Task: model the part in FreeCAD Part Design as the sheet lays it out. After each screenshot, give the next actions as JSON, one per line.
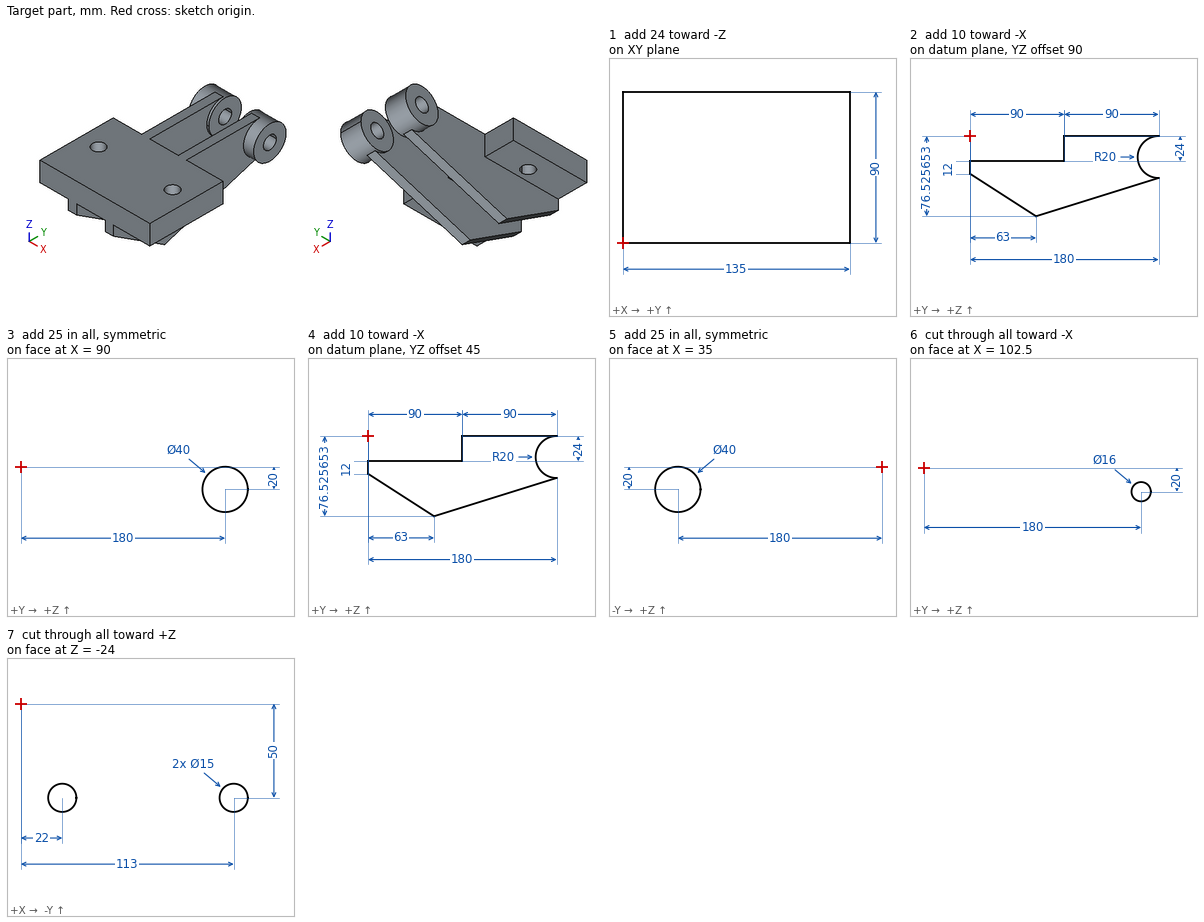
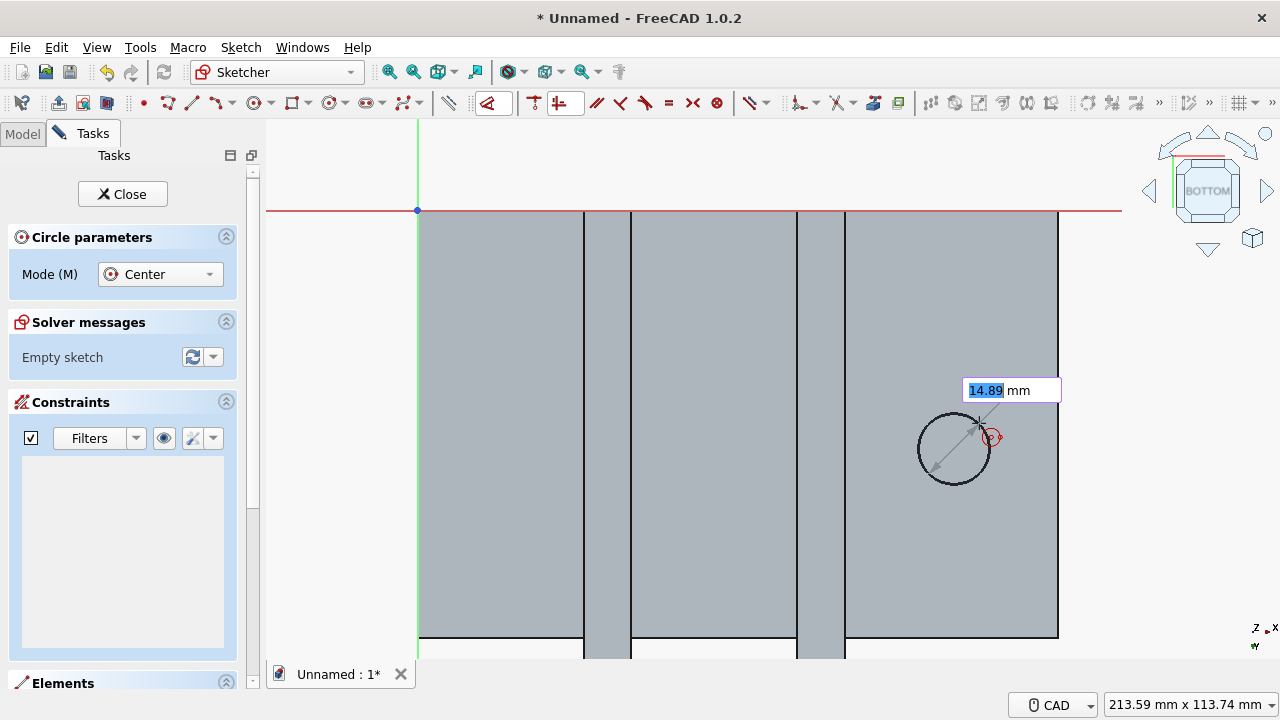
{"action": "type", "text": "15"}
{"action": "key", "text": "Return"}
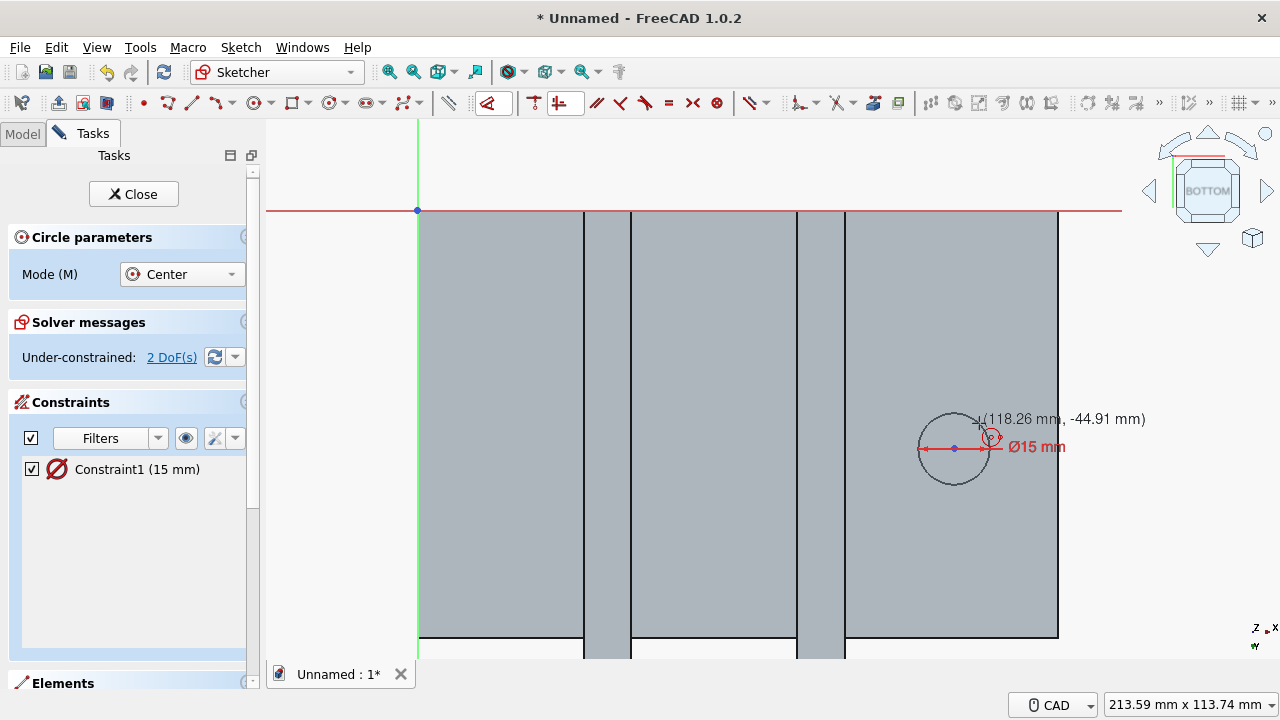
{"action": "left_click", "coordinate": [522, 448]}
{"action": "mouse_move", "coordinate": [547, 423]}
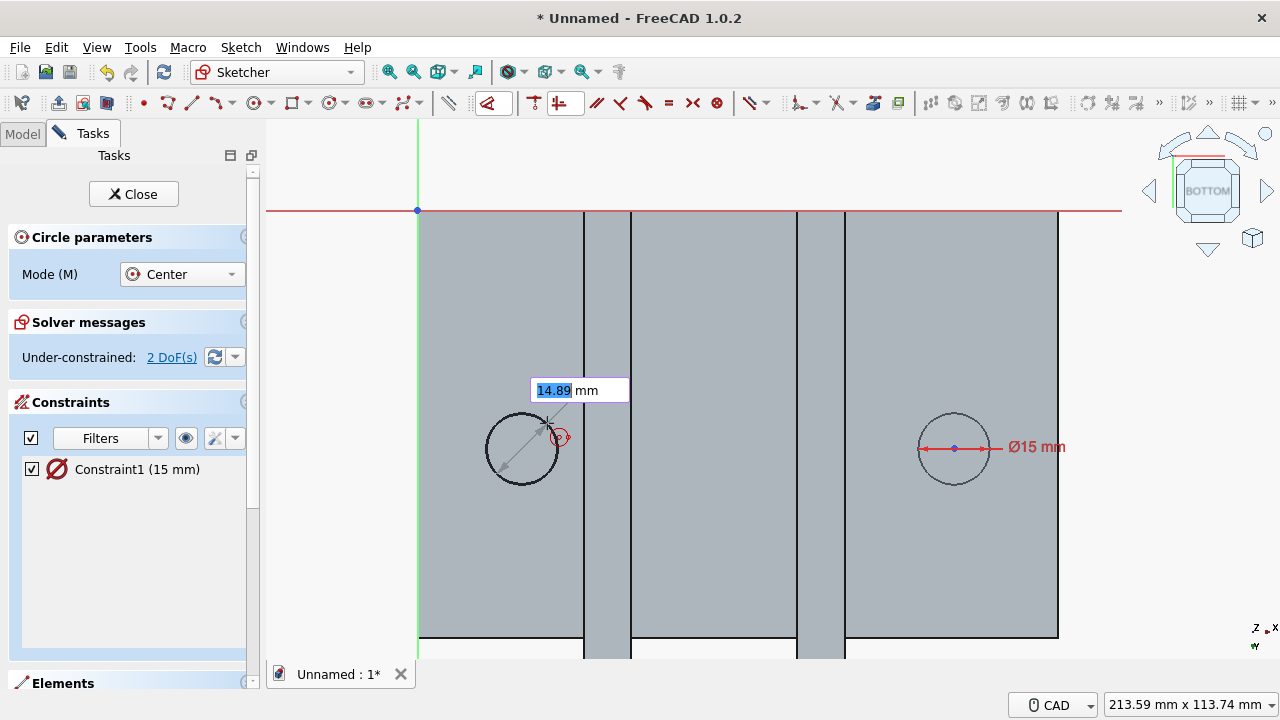
{"action": "type", "text": "15"}
{"action": "key", "text": "Return"}
{"action": "key", "text": "Escape"}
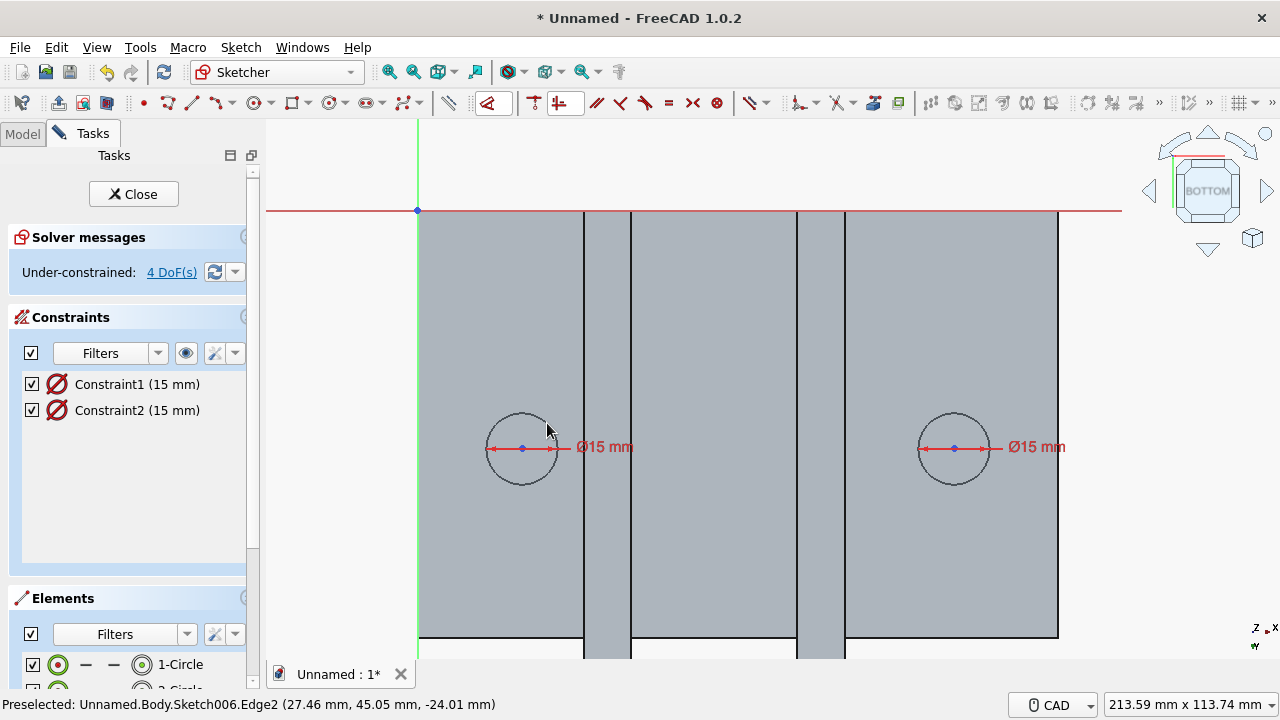
{"action": "left_click", "coordinate": [954, 449]}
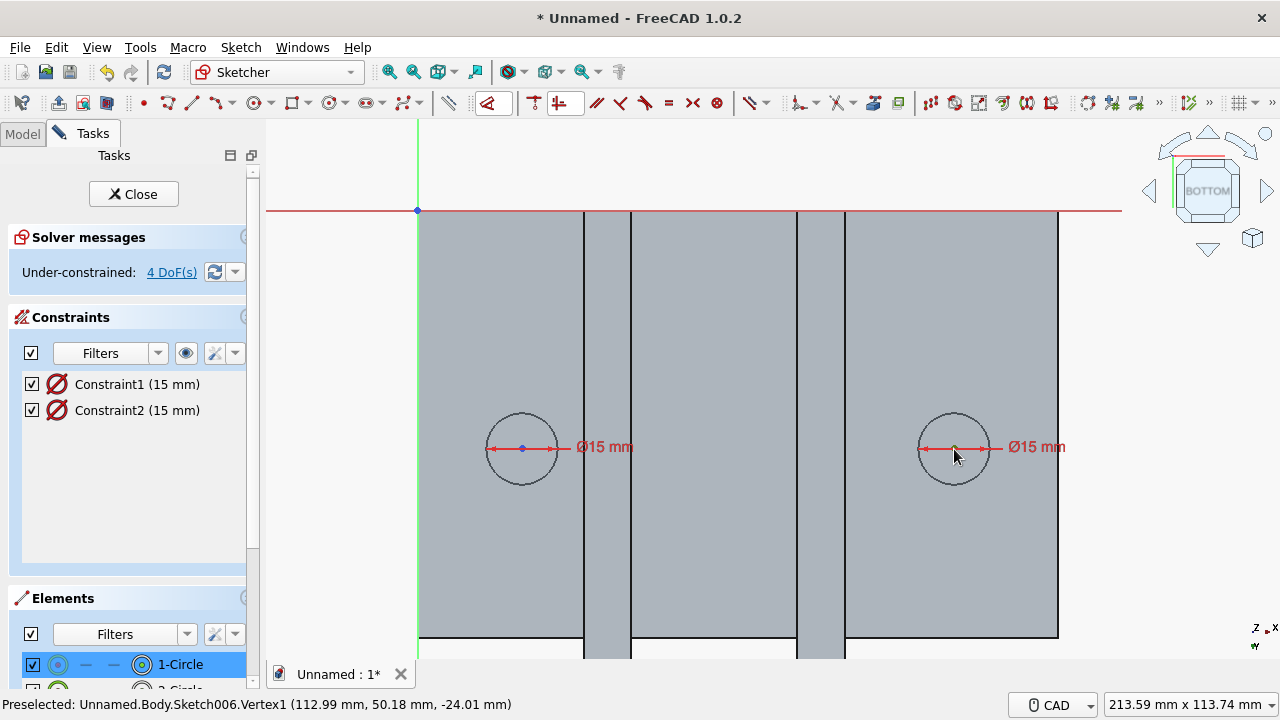
{"action": "left_click", "coordinate": [522, 449]}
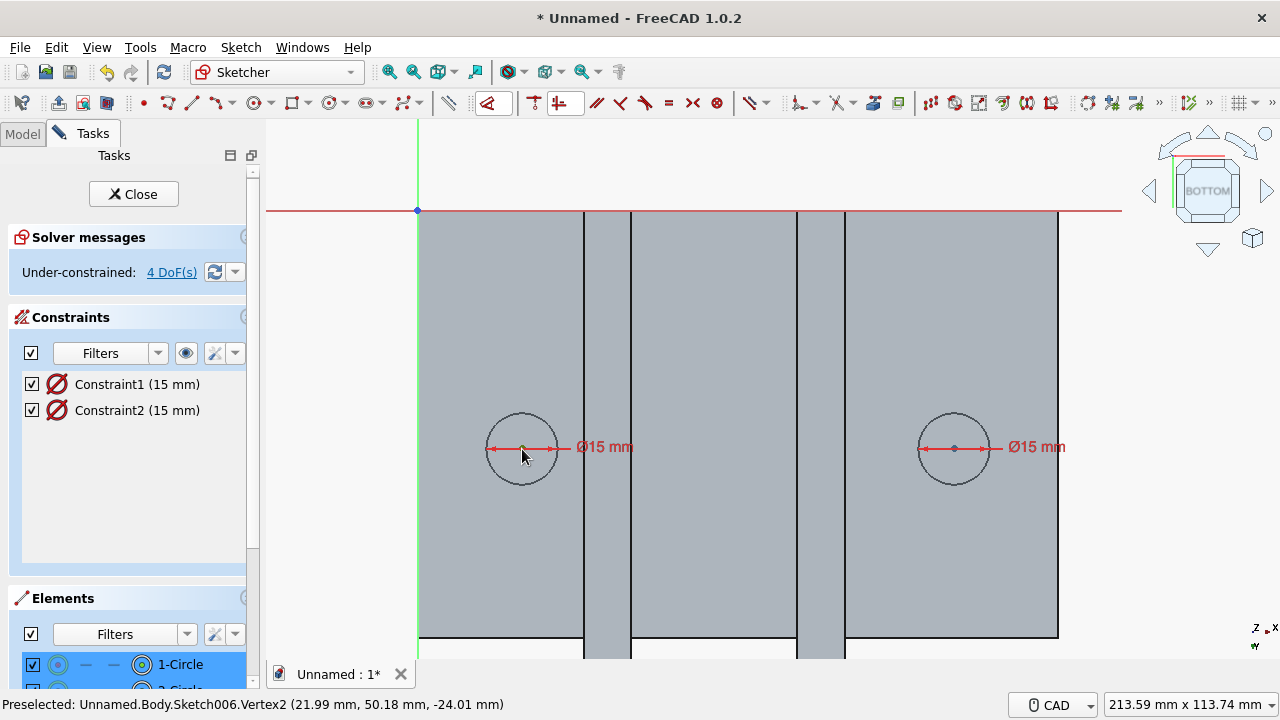
{"action": "left_click", "coordinate": [578, 104]}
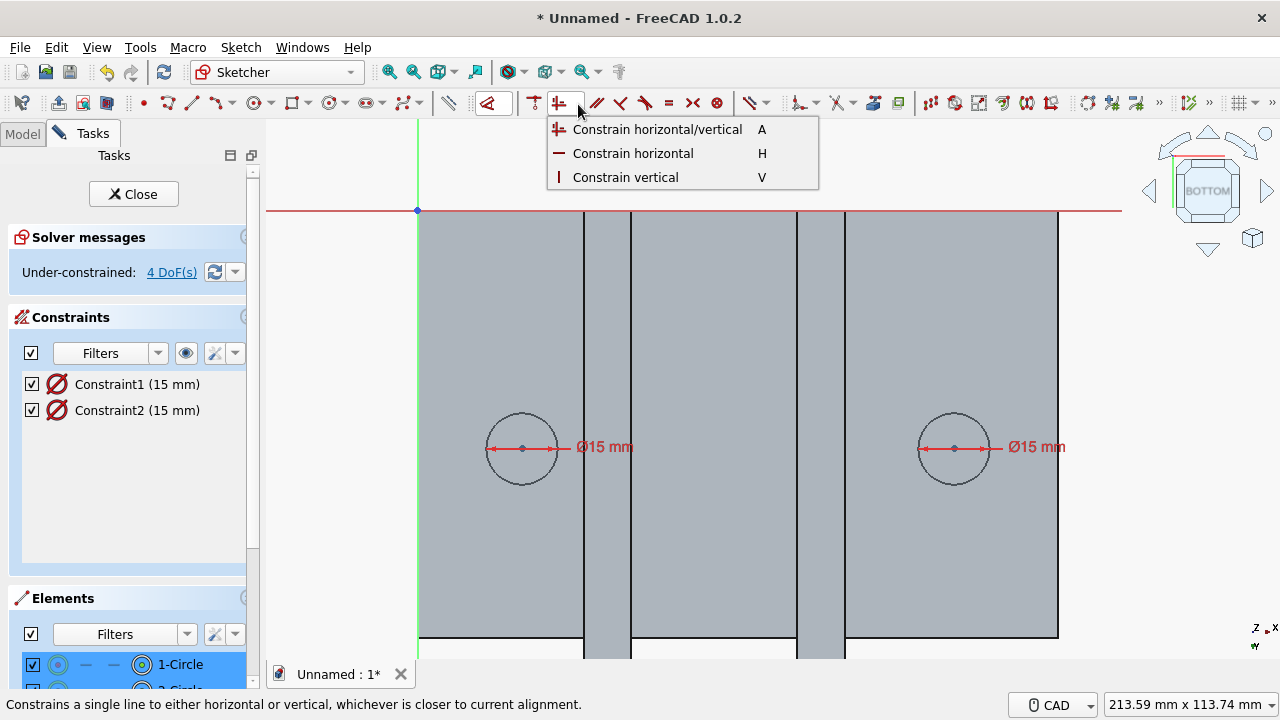
{"action": "left_click", "coordinate": [683, 153]}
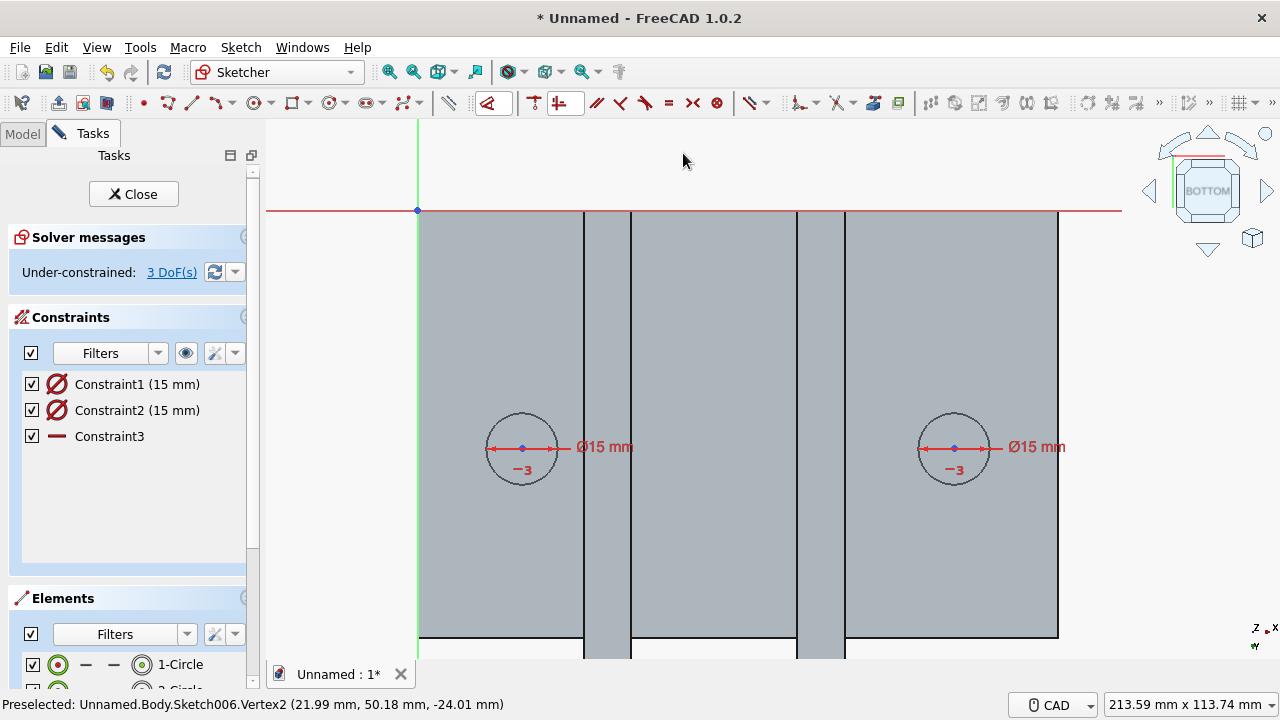
{"action": "left_click", "coordinate": [954, 449]}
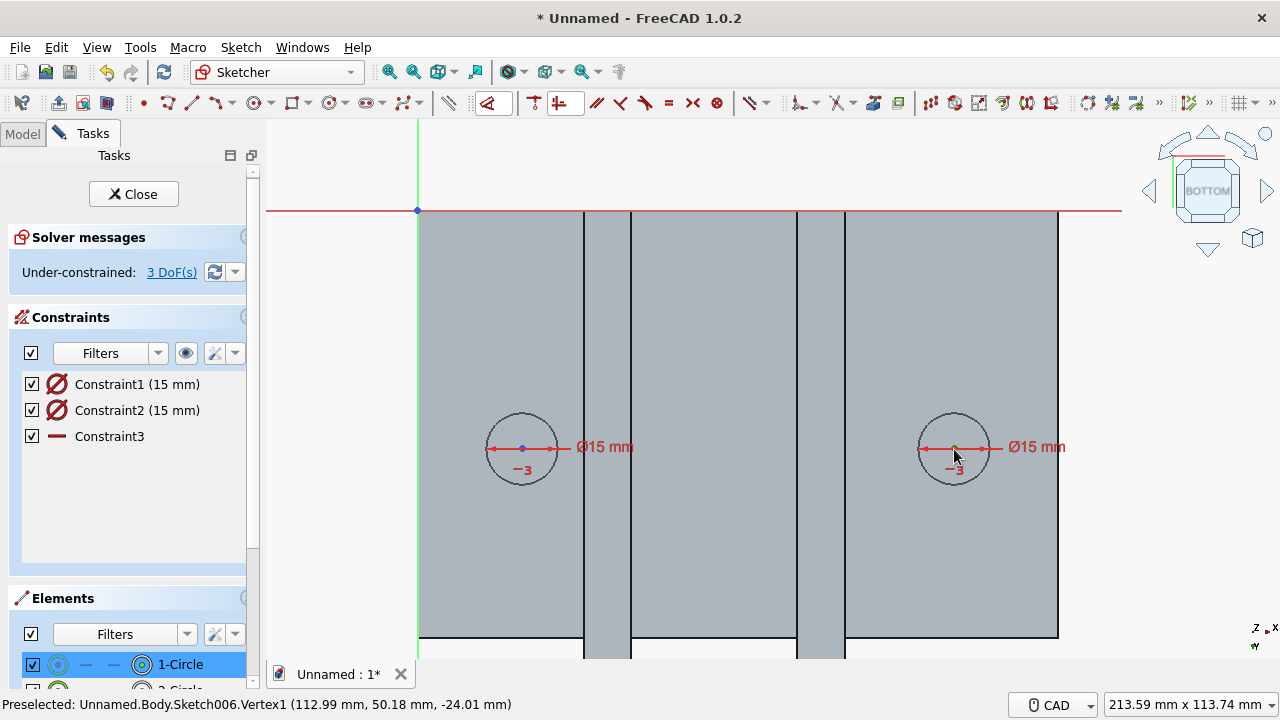
{"action": "key", "text": "i"}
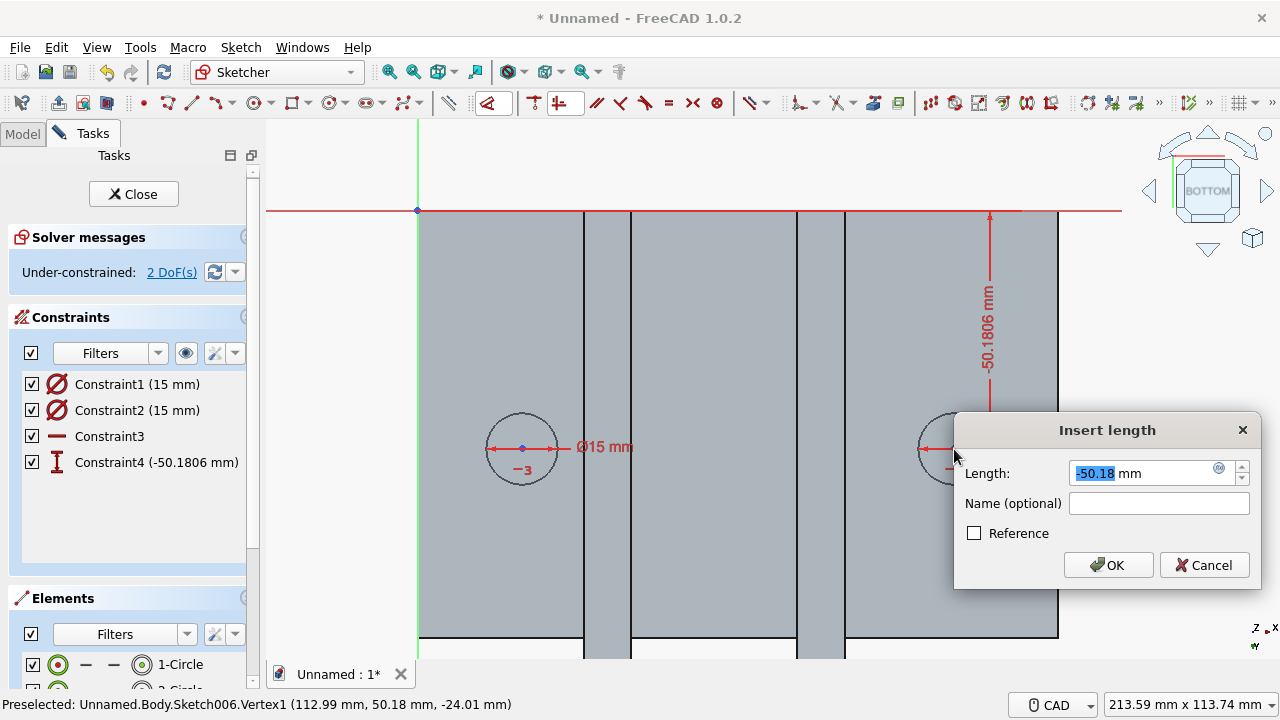
{"action": "type", "text": "-50"}
{"action": "key", "text": "Return"}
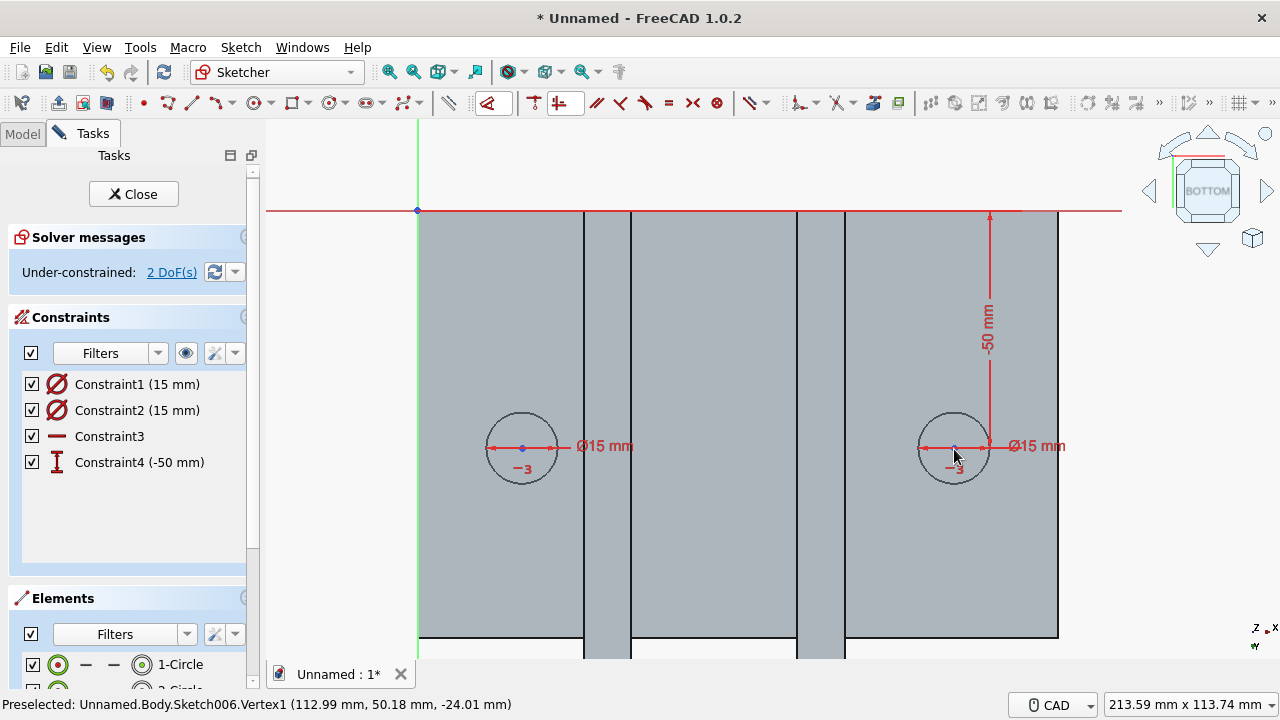
{"action": "left_click", "coordinate": [522, 448]}